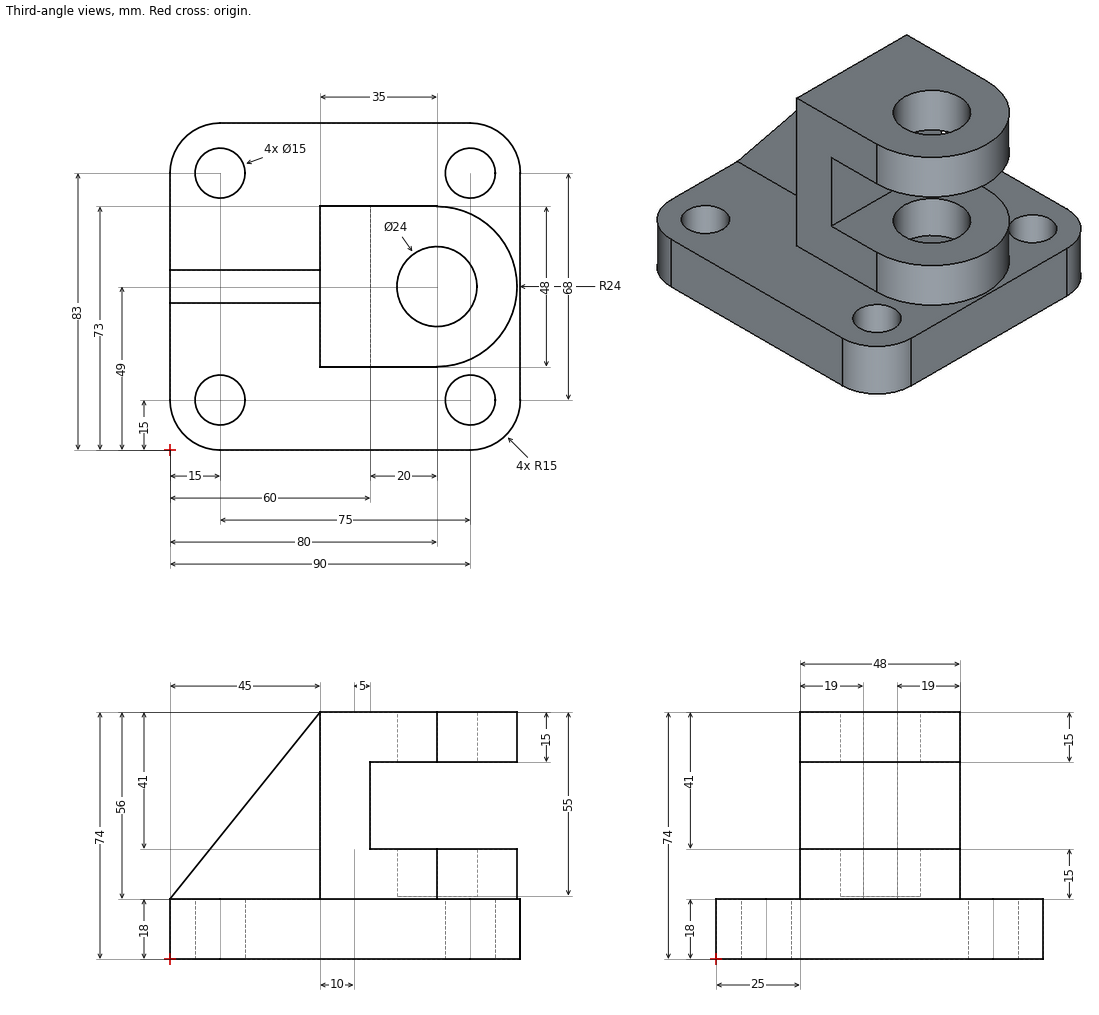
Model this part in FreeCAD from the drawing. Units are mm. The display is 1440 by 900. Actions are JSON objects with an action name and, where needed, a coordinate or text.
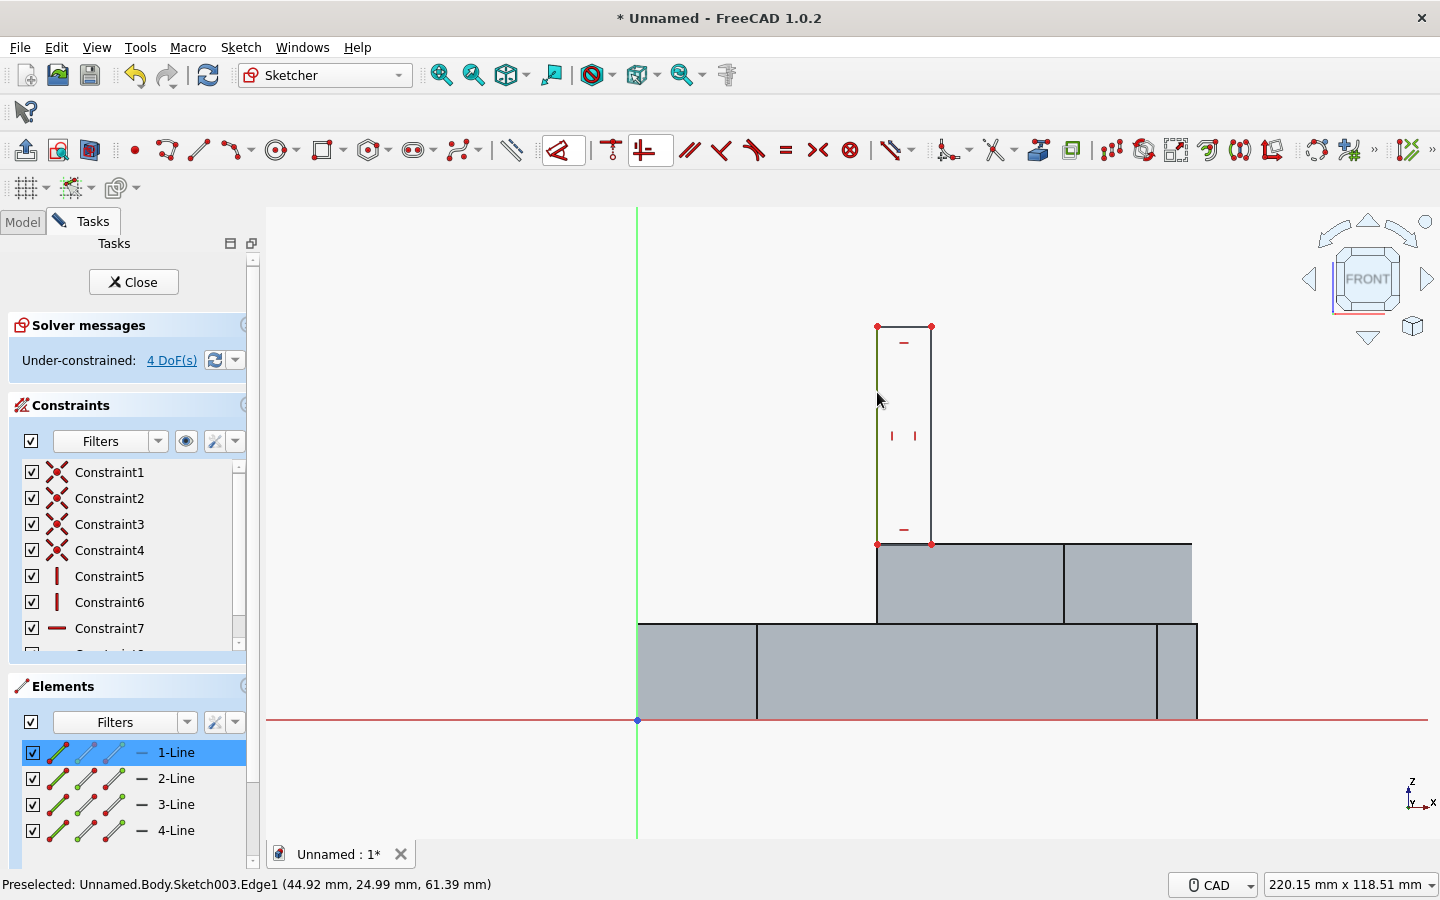
{"action": "key", "text": "i"}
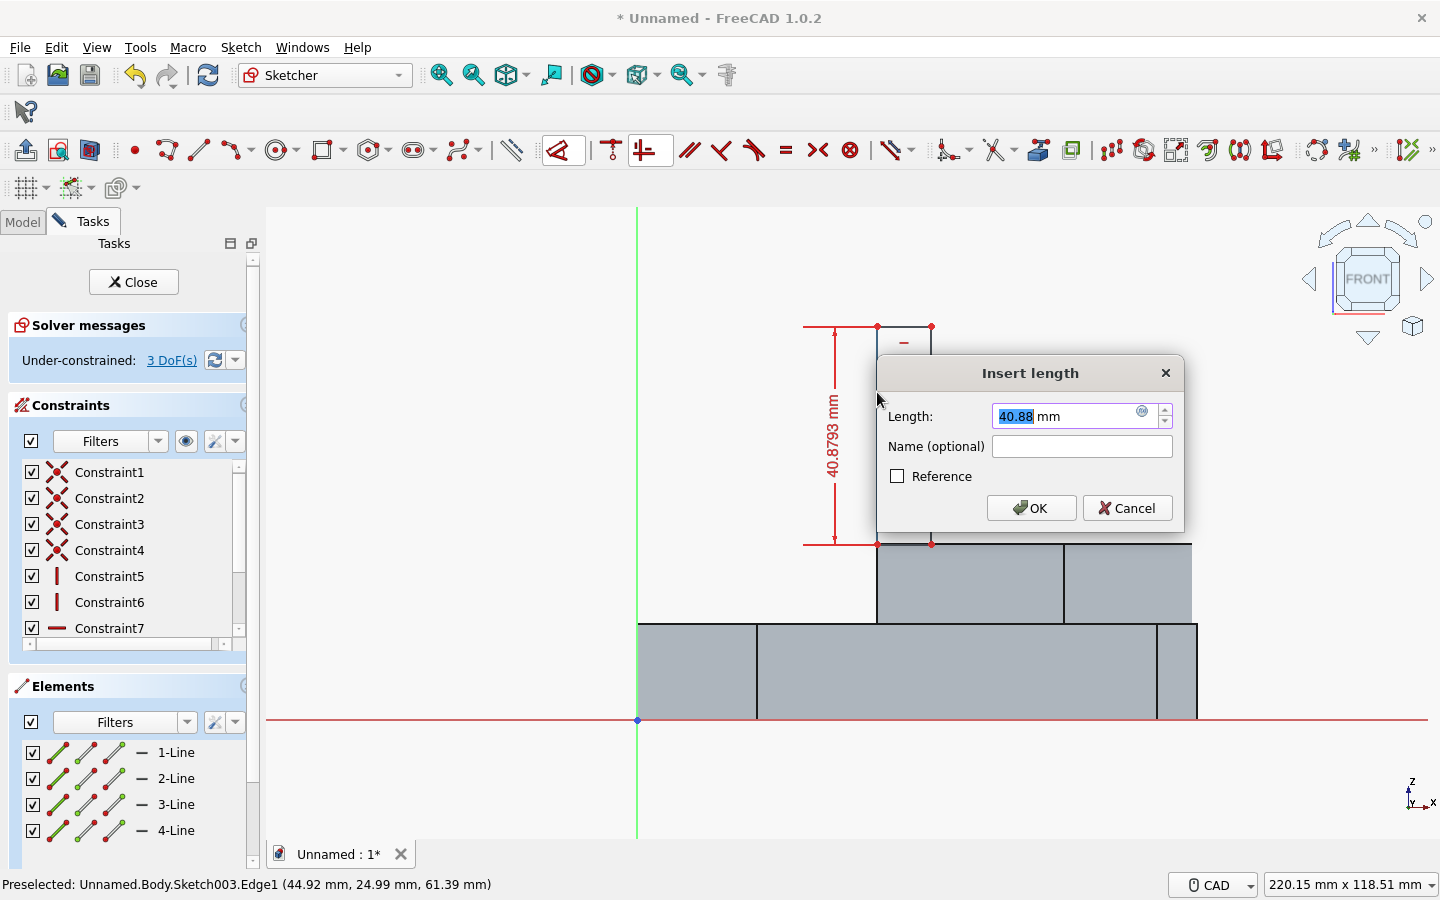
{"action": "type", "text": "41"}
{"action": "key", "text": "Return"}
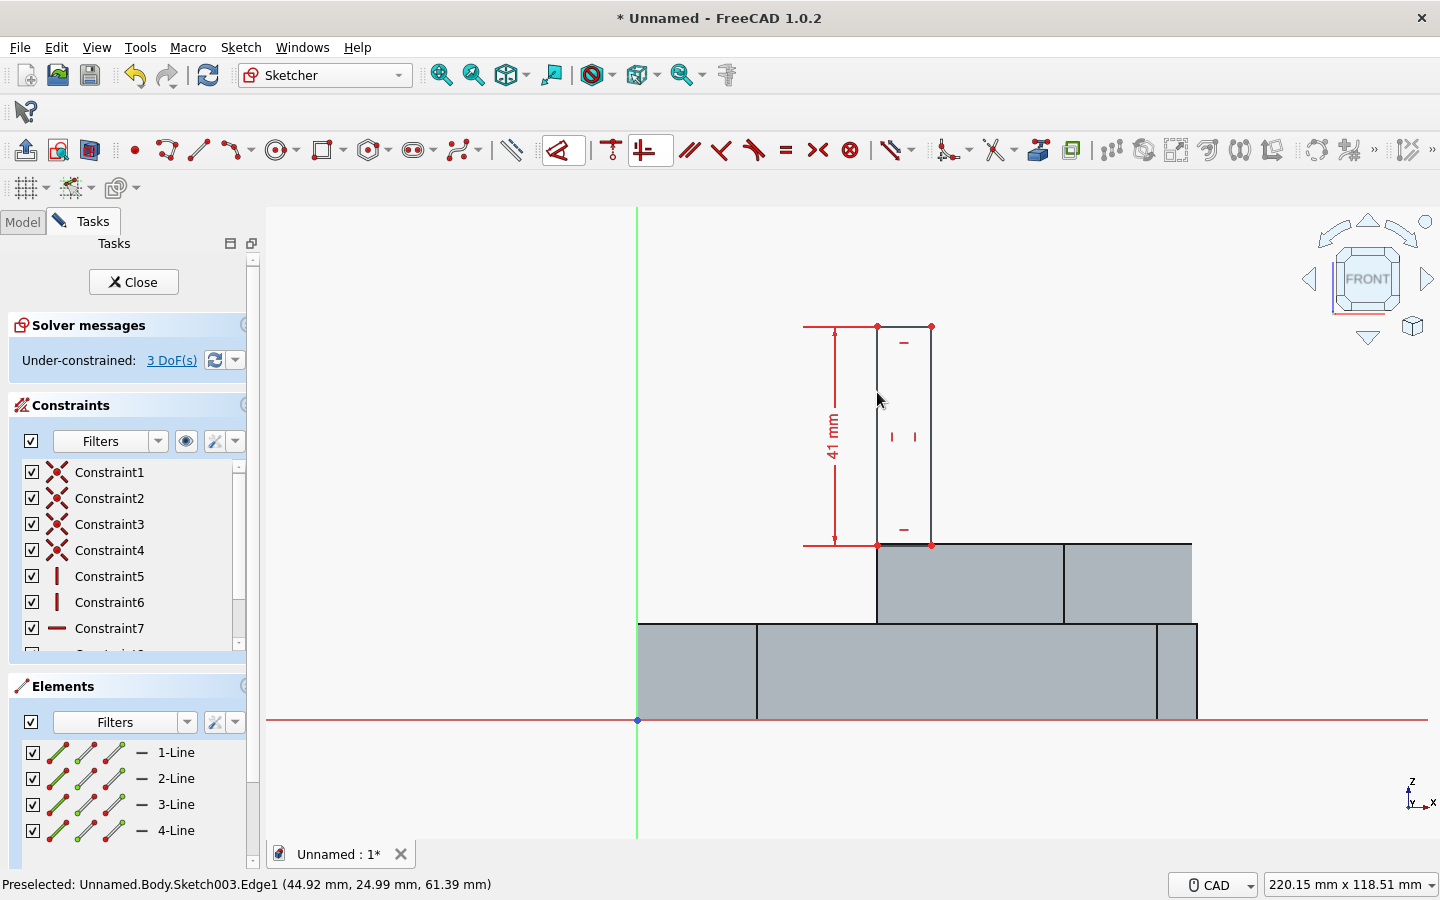
{"action": "left_click", "coordinate": [893, 546]}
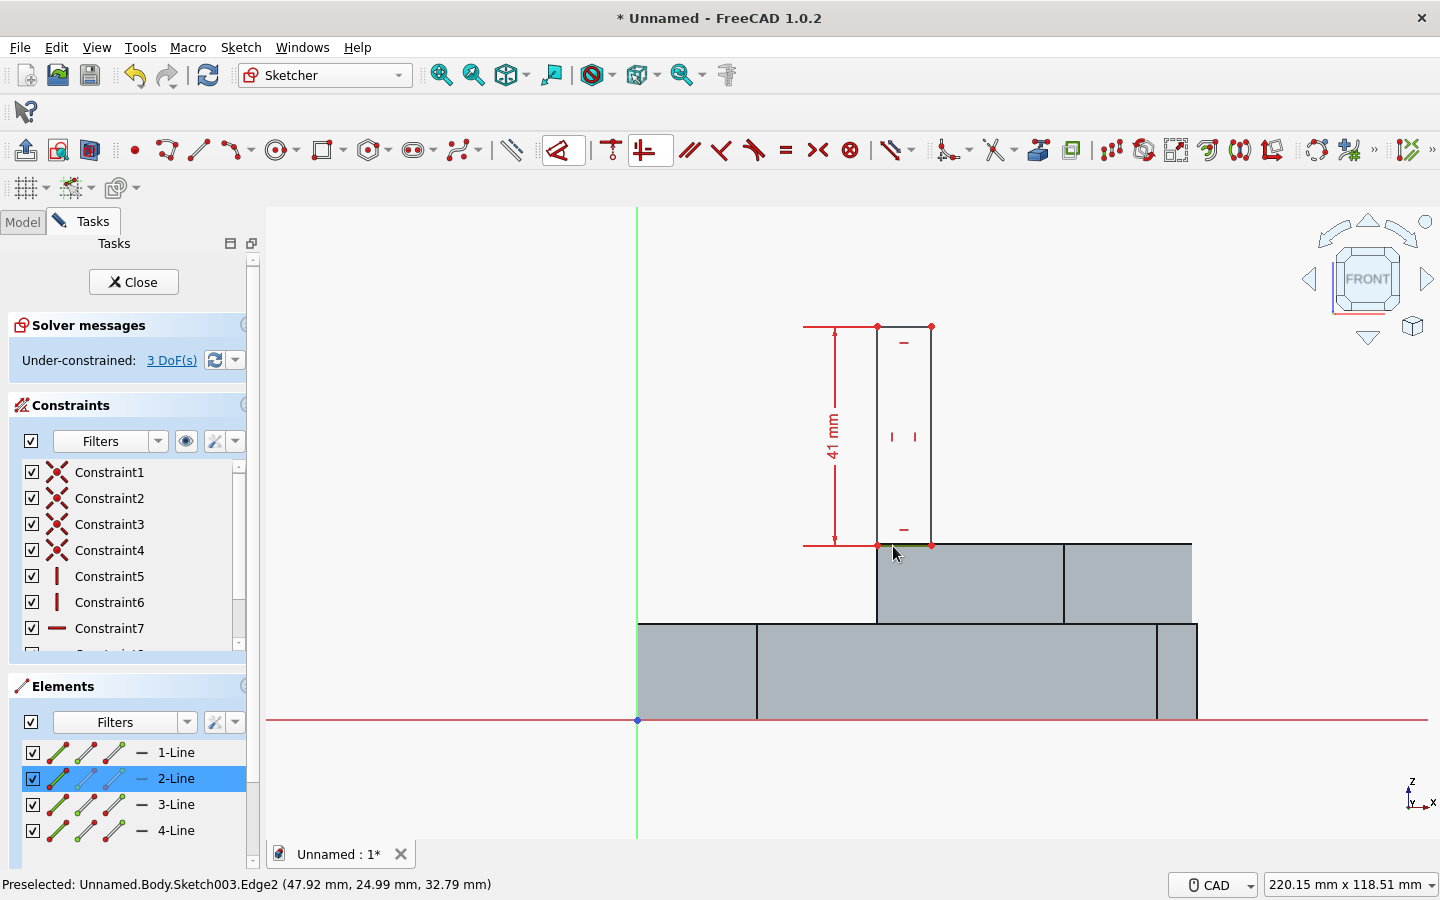
{"action": "left_click", "coordinate": [580, 150]}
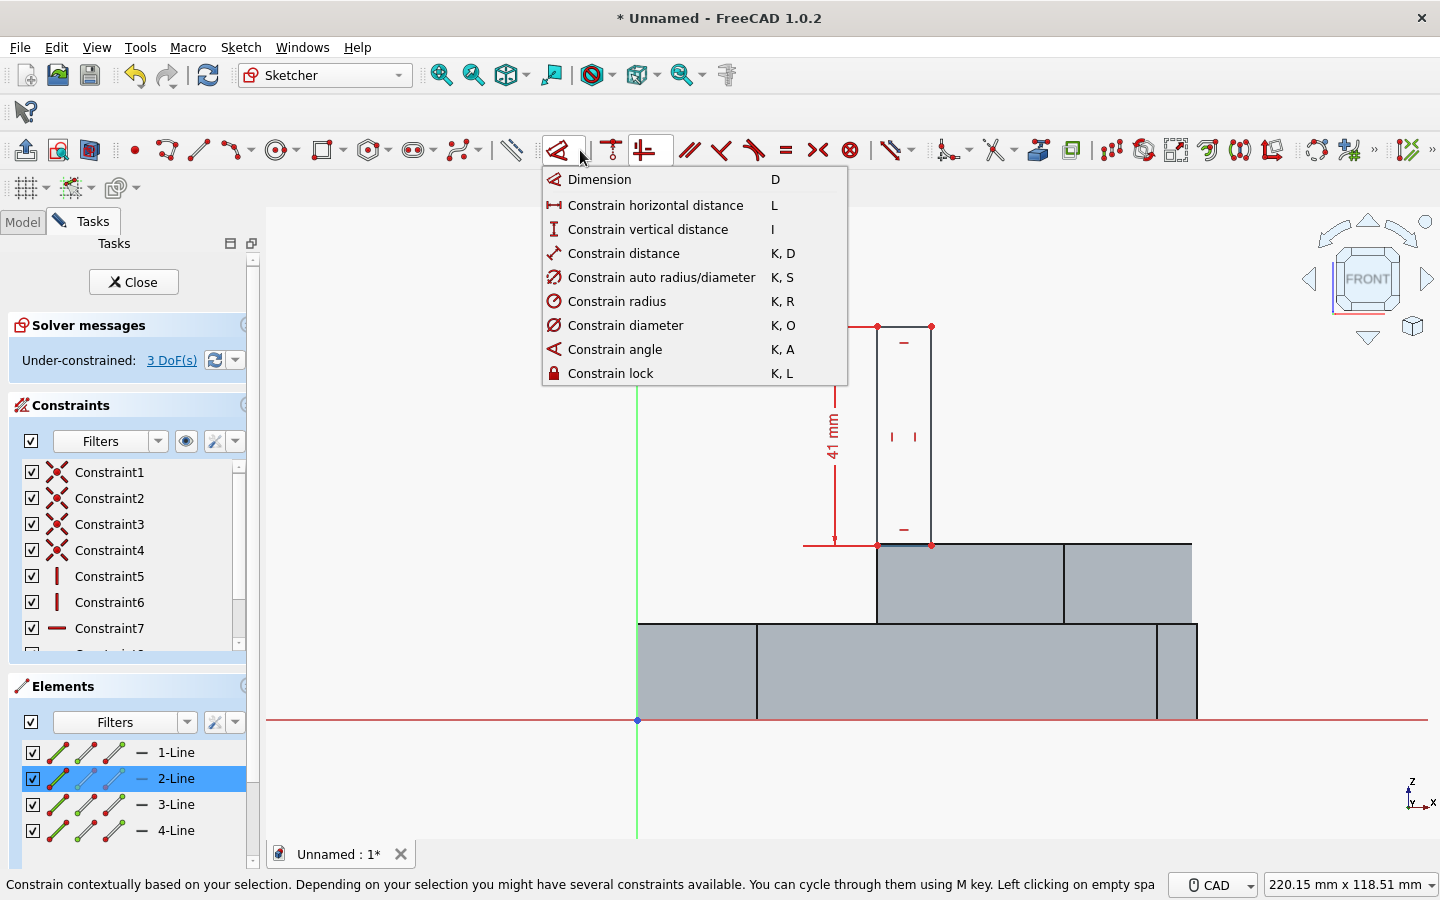
{"action": "left_click", "coordinate": [695, 205]}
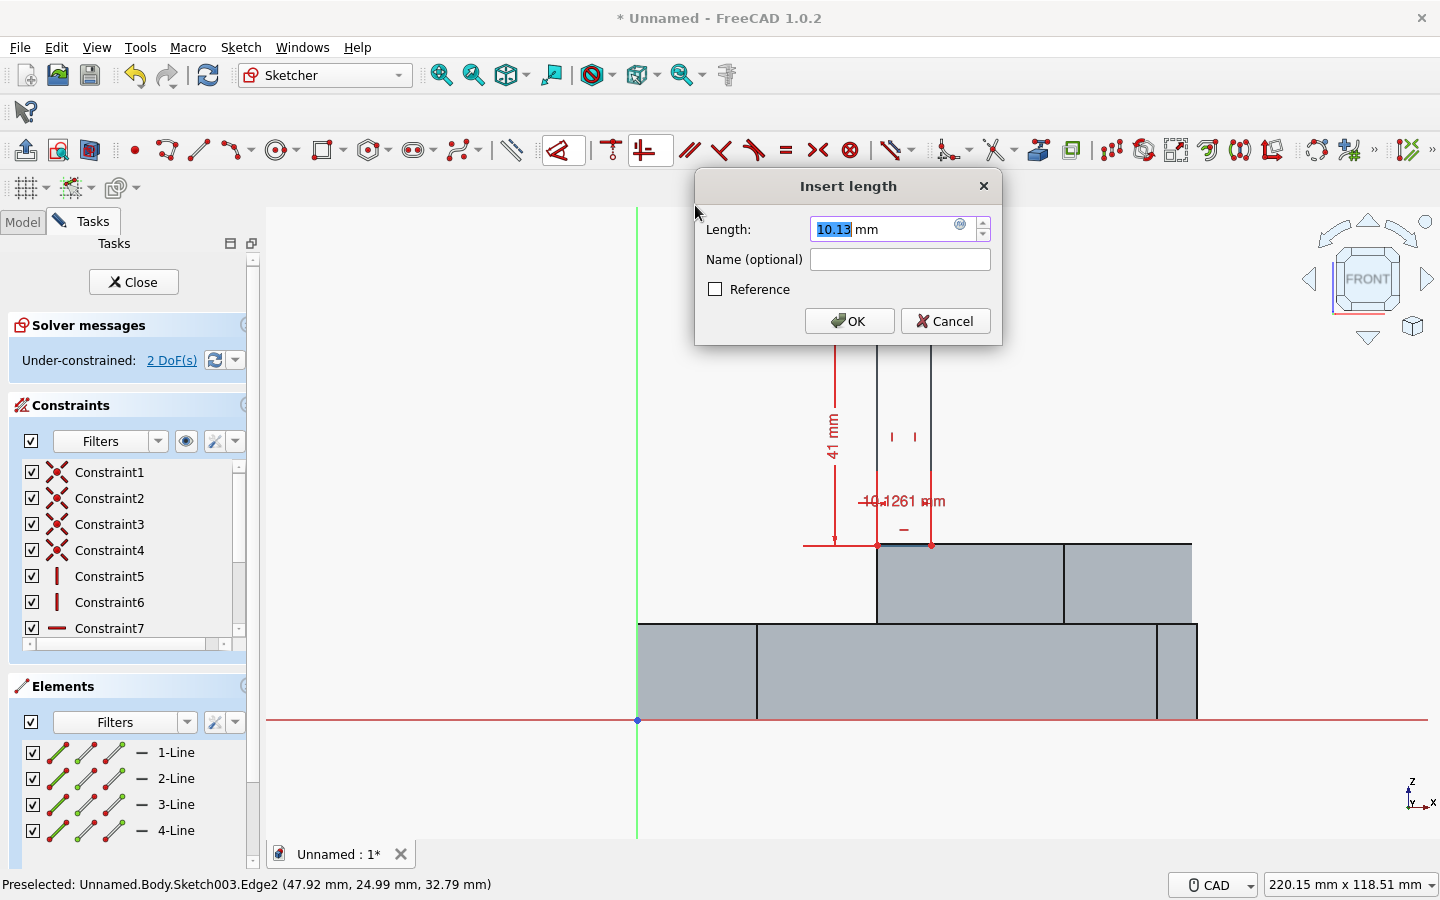
{"action": "type", "text": "10"}
{"action": "key", "text": "Return"}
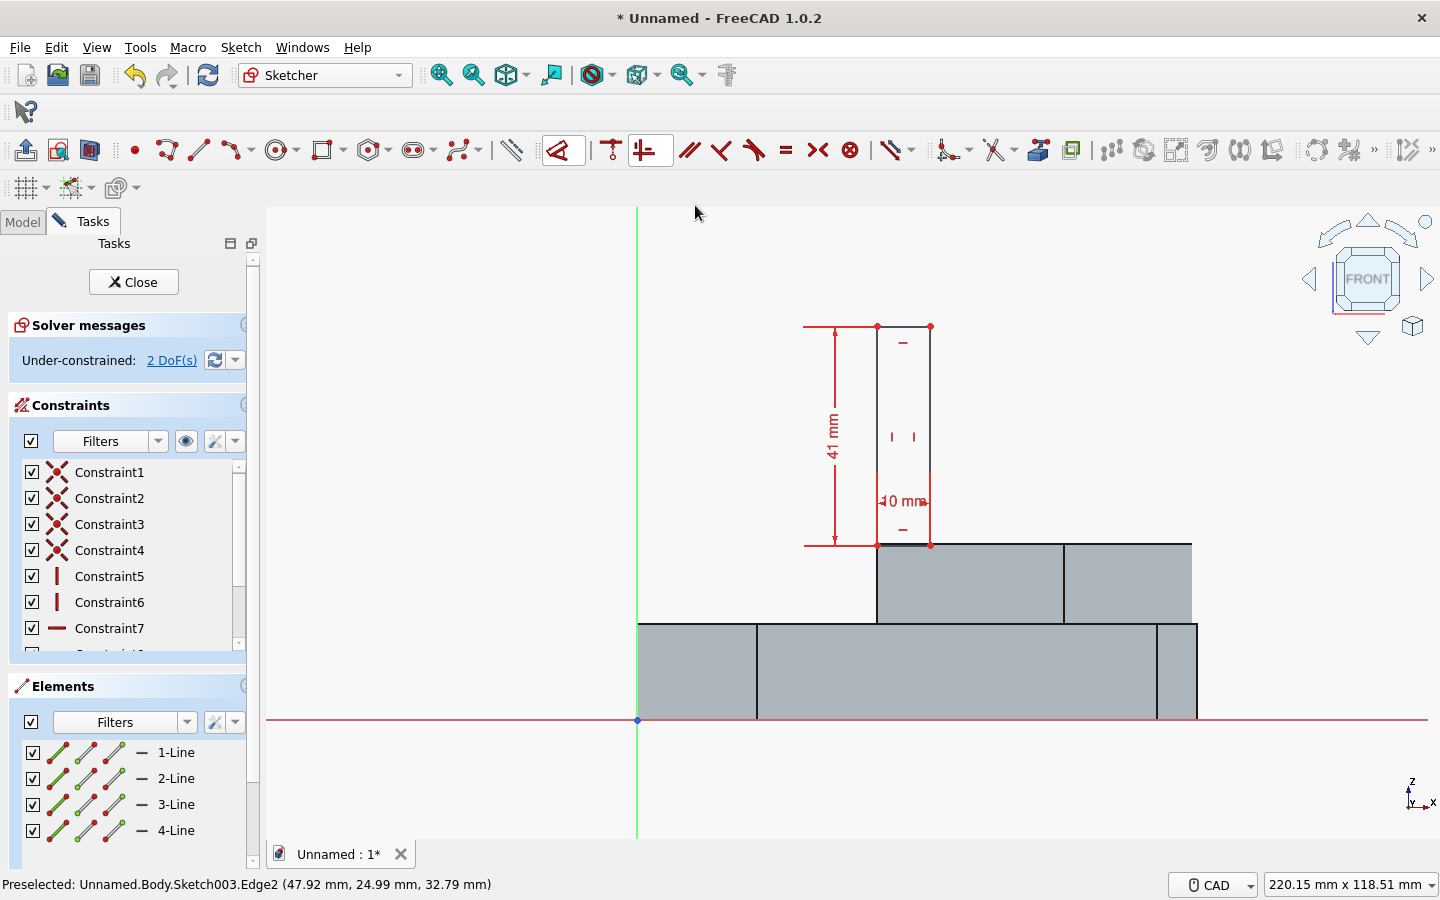
{"action": "left_click", "coordinate": [877, 327]}